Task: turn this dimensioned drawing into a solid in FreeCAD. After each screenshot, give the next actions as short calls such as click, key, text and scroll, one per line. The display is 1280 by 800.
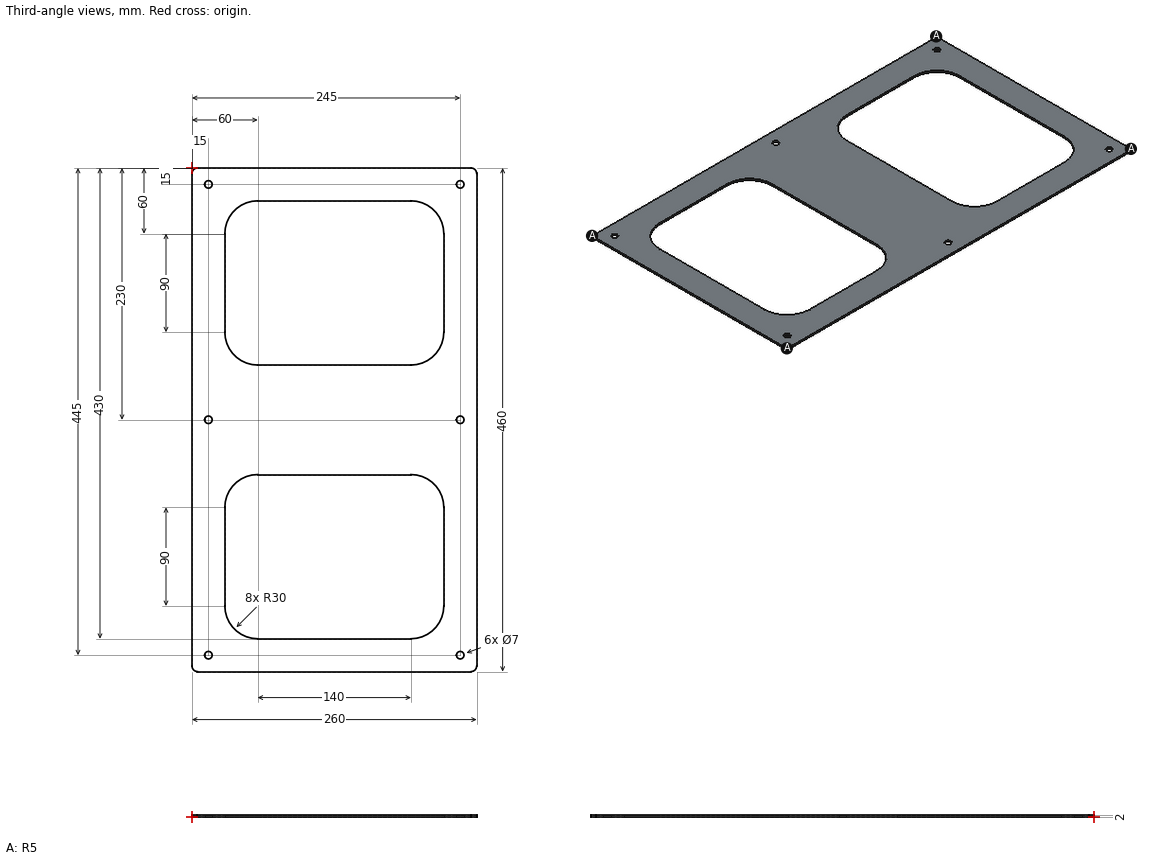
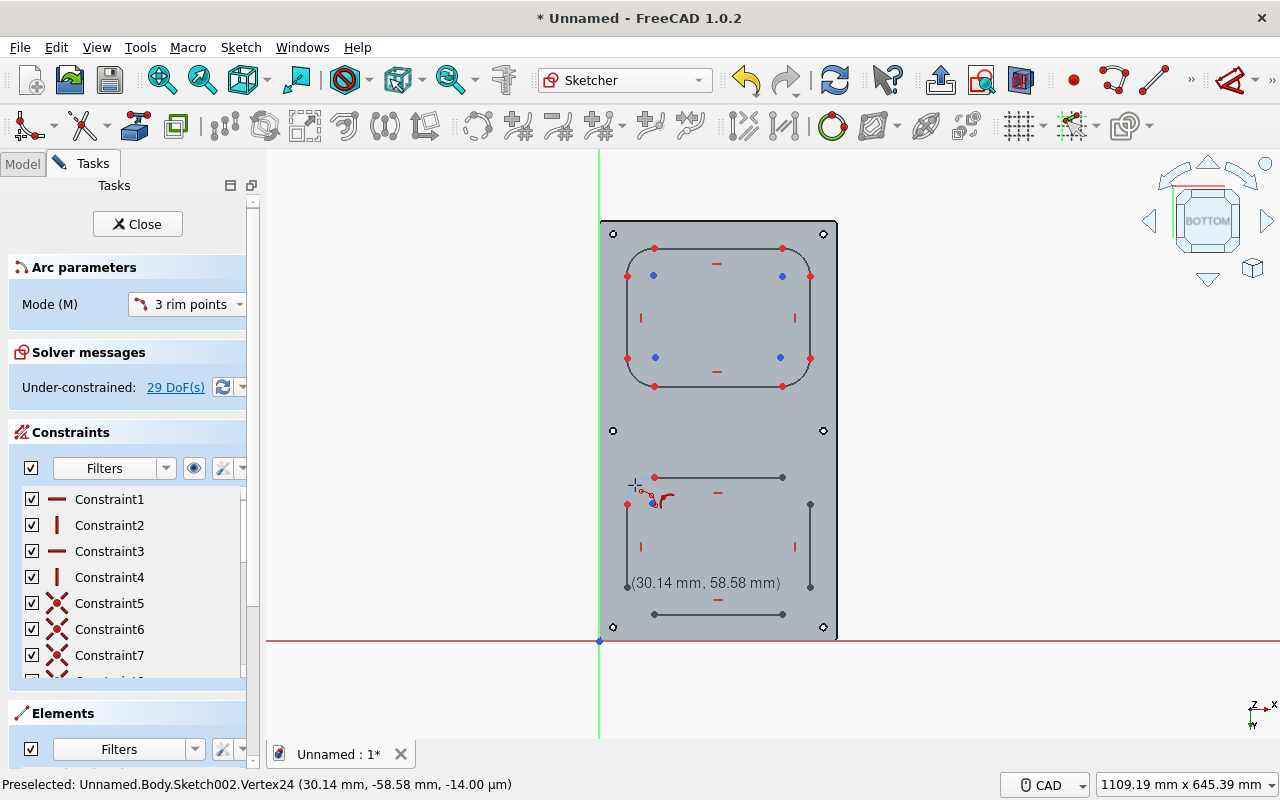
click(654, 615)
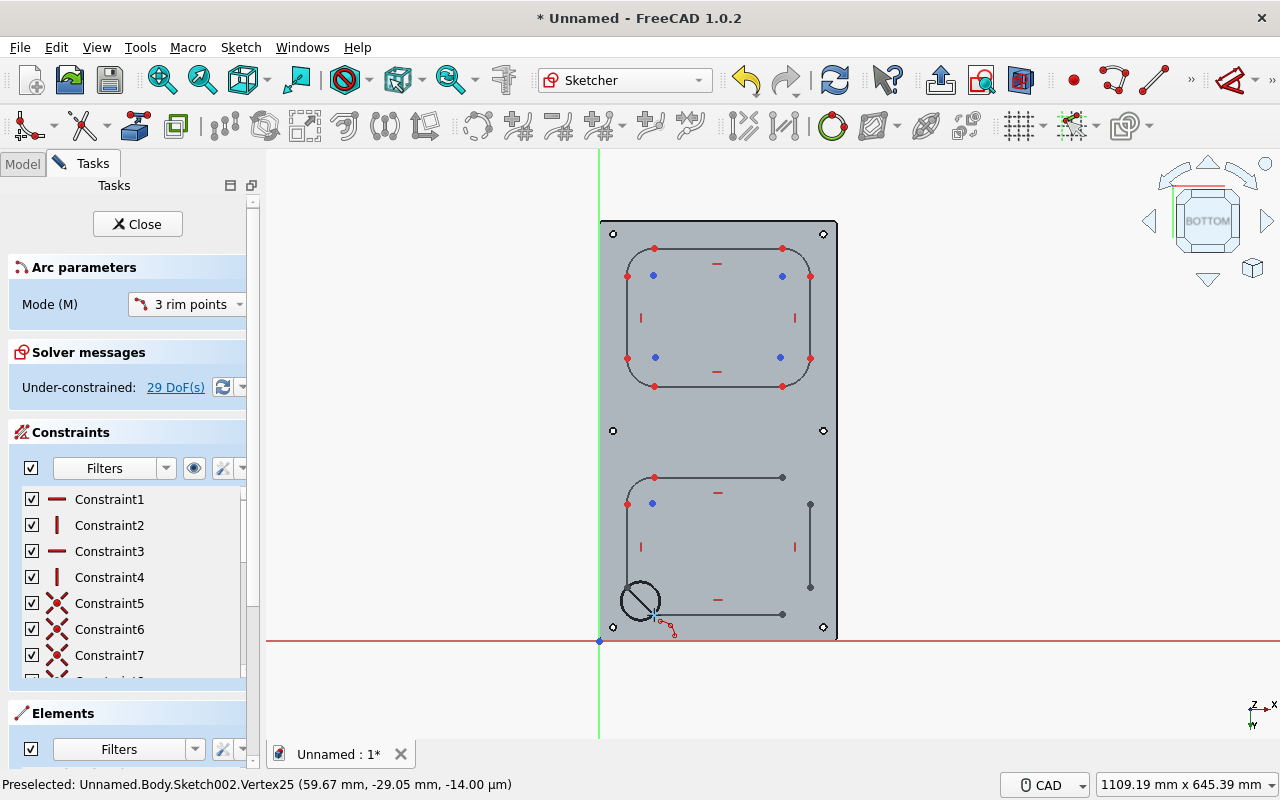
scroll(635, 606, up, 4)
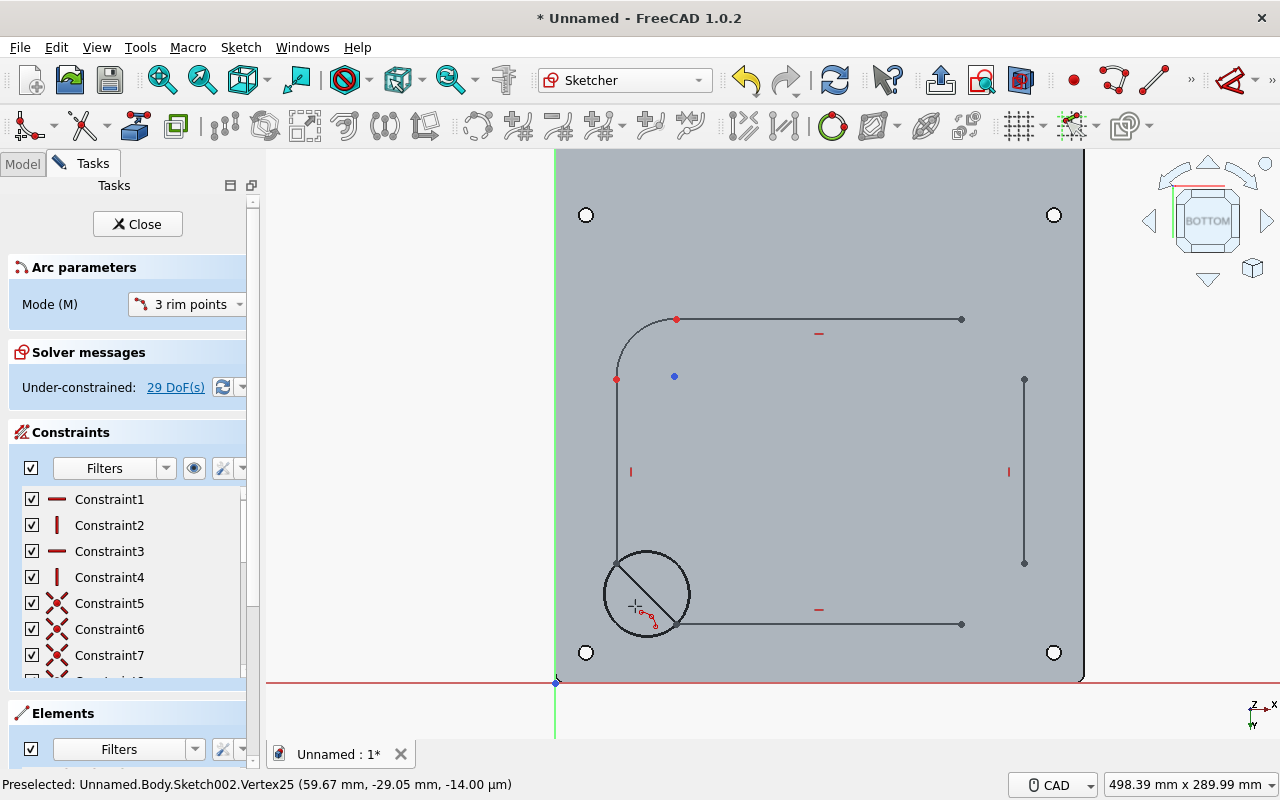
click(634, 604)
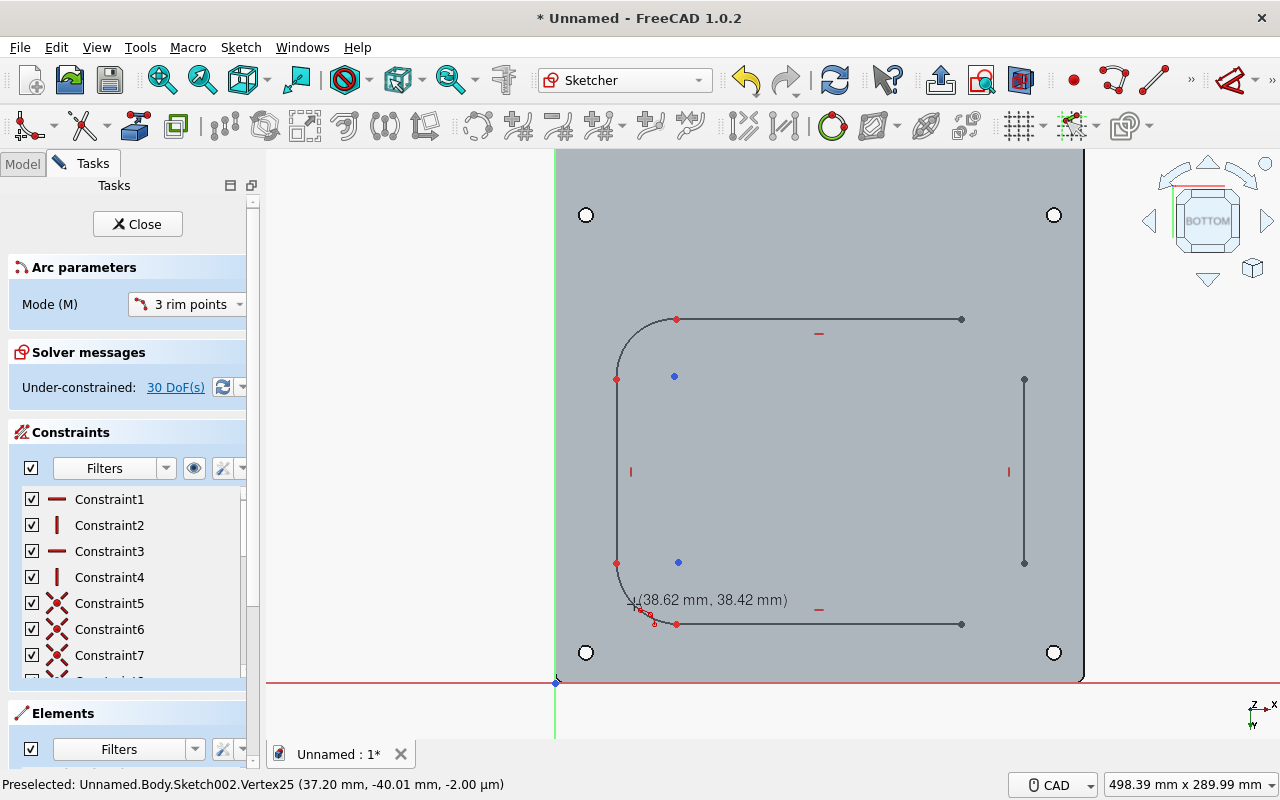
click(962, 624)
click(1024, 564)
click(1006, 604)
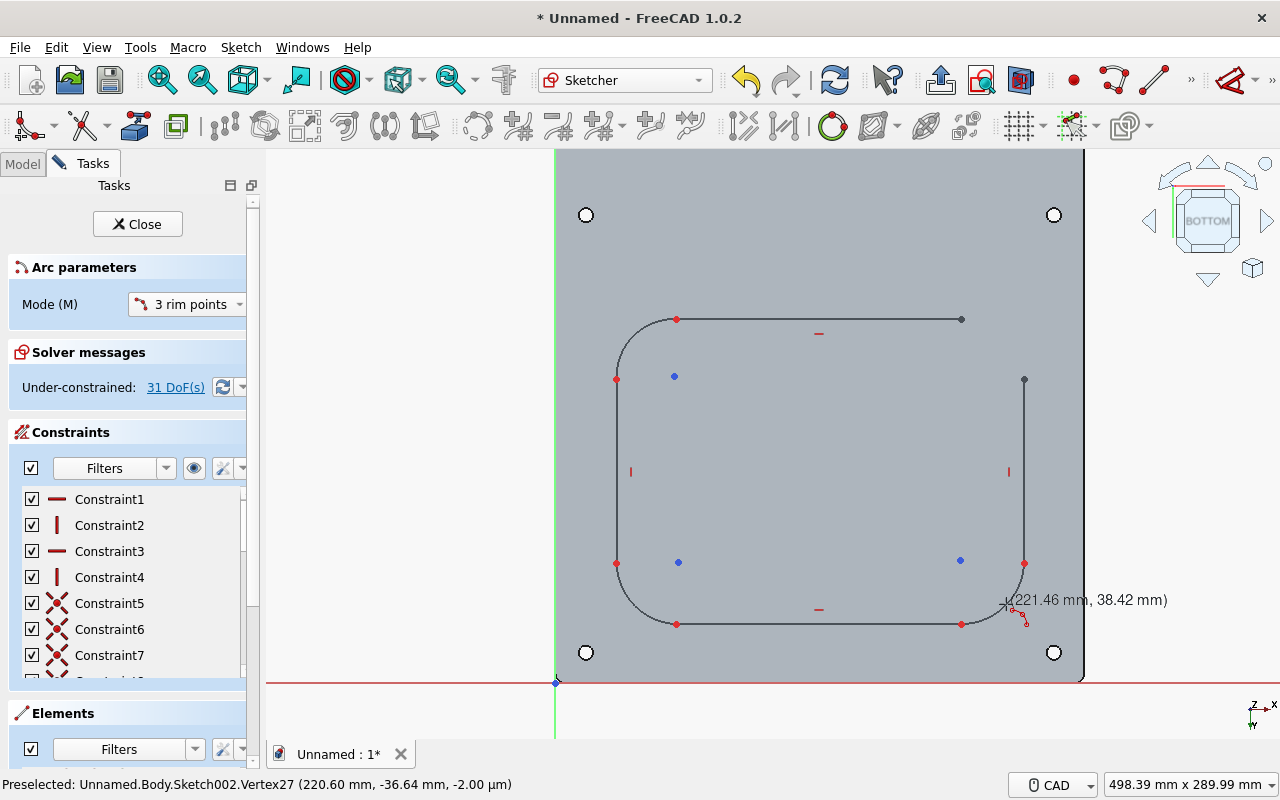
click(1024, 379)
click(962, 319)
click(1006, 335)
key(Escape)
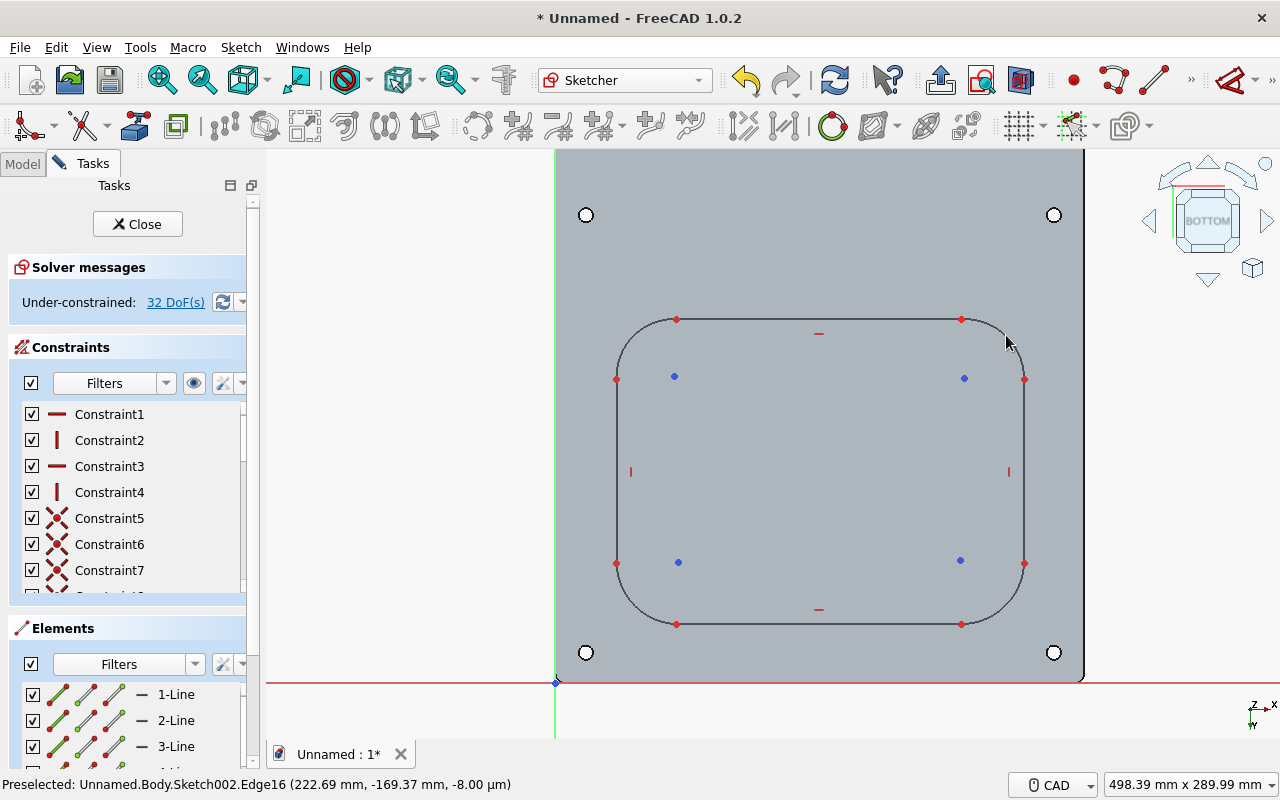
scroll(635, 606, down, 4)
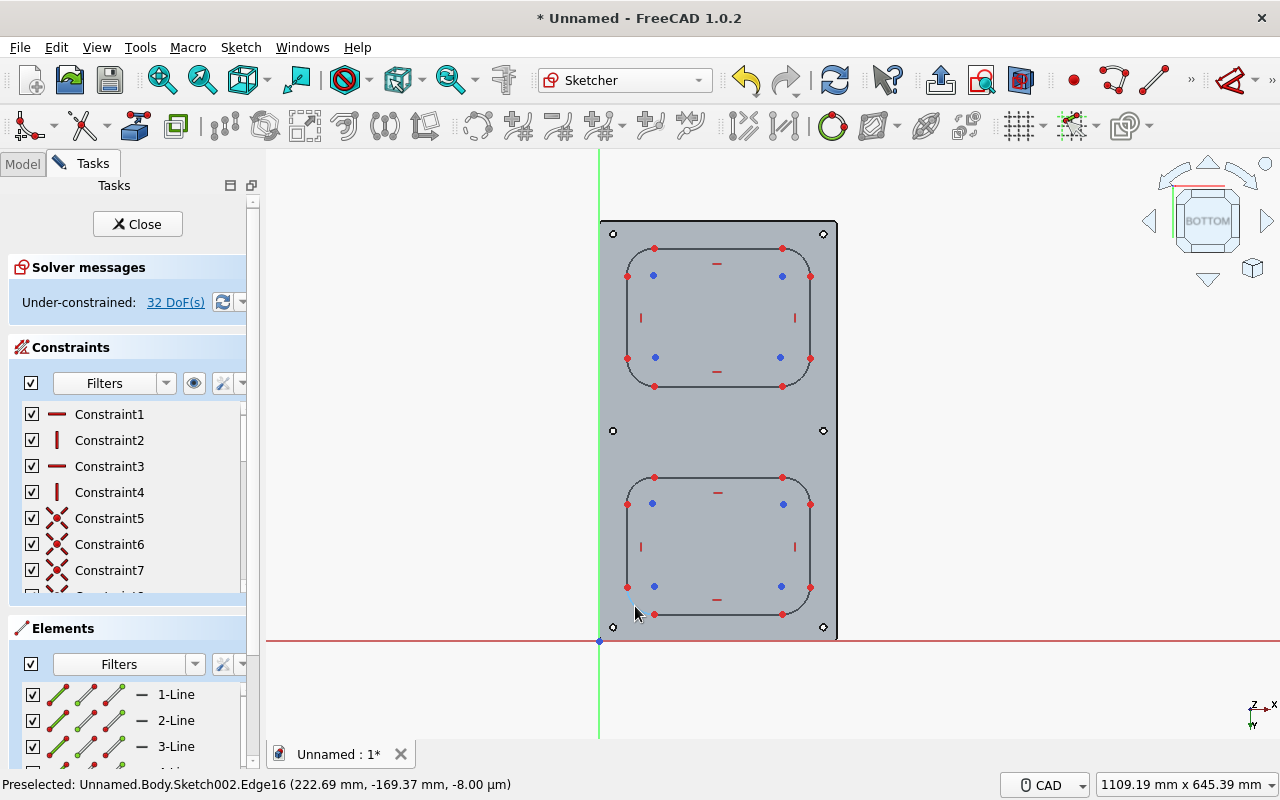
click(744, 249)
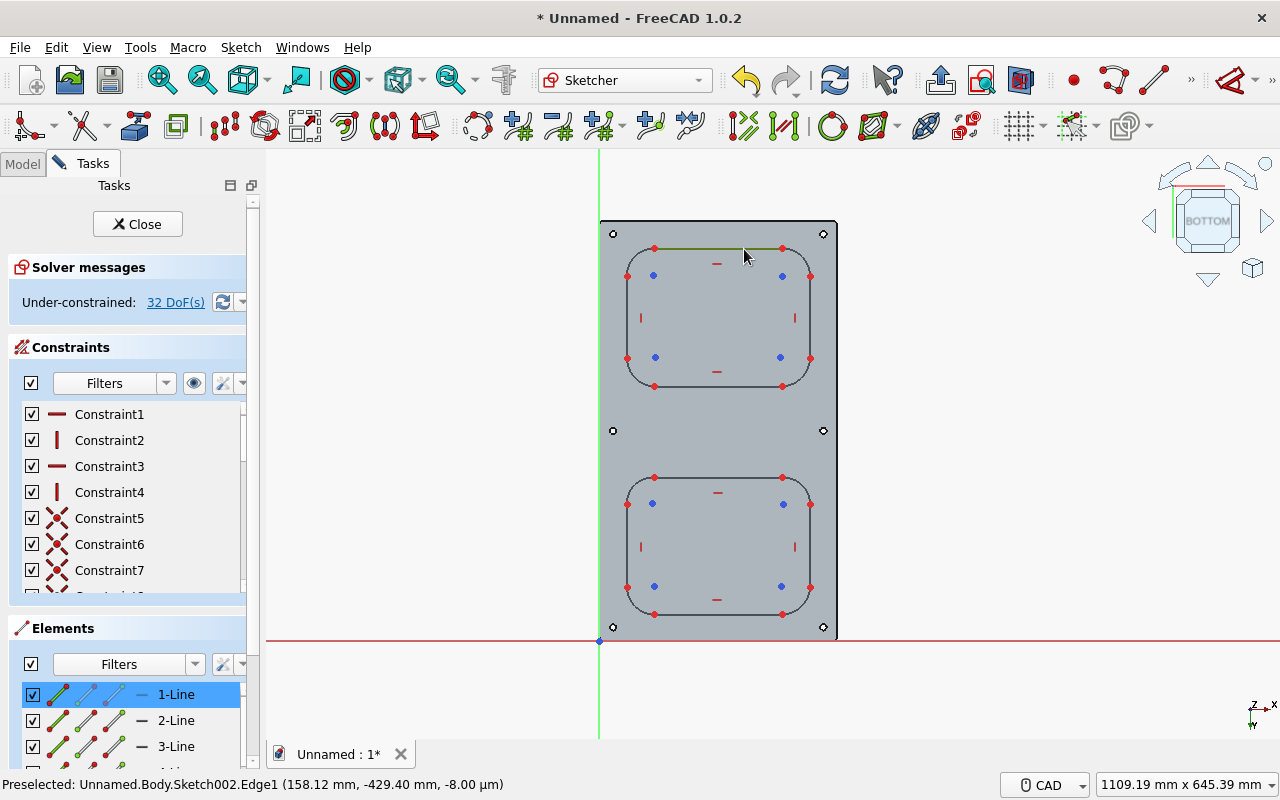
click(641, 252)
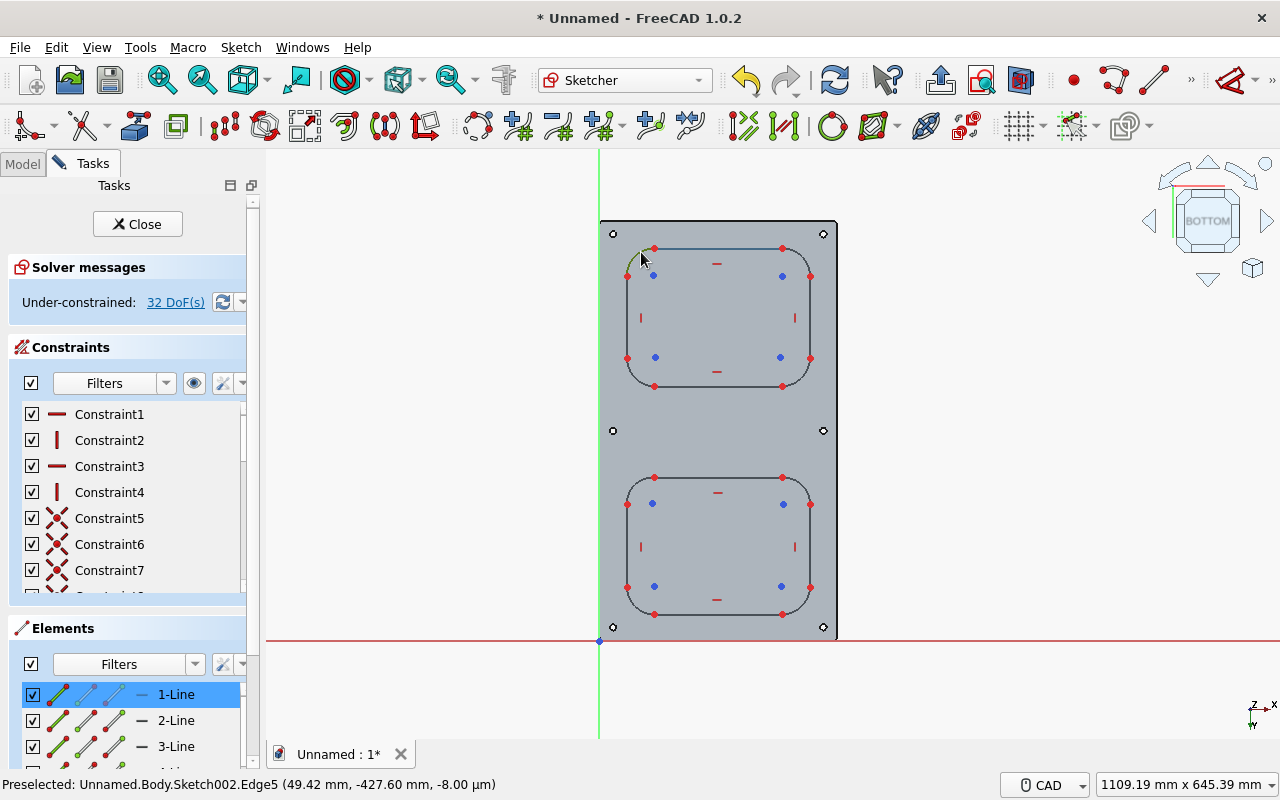
key(t)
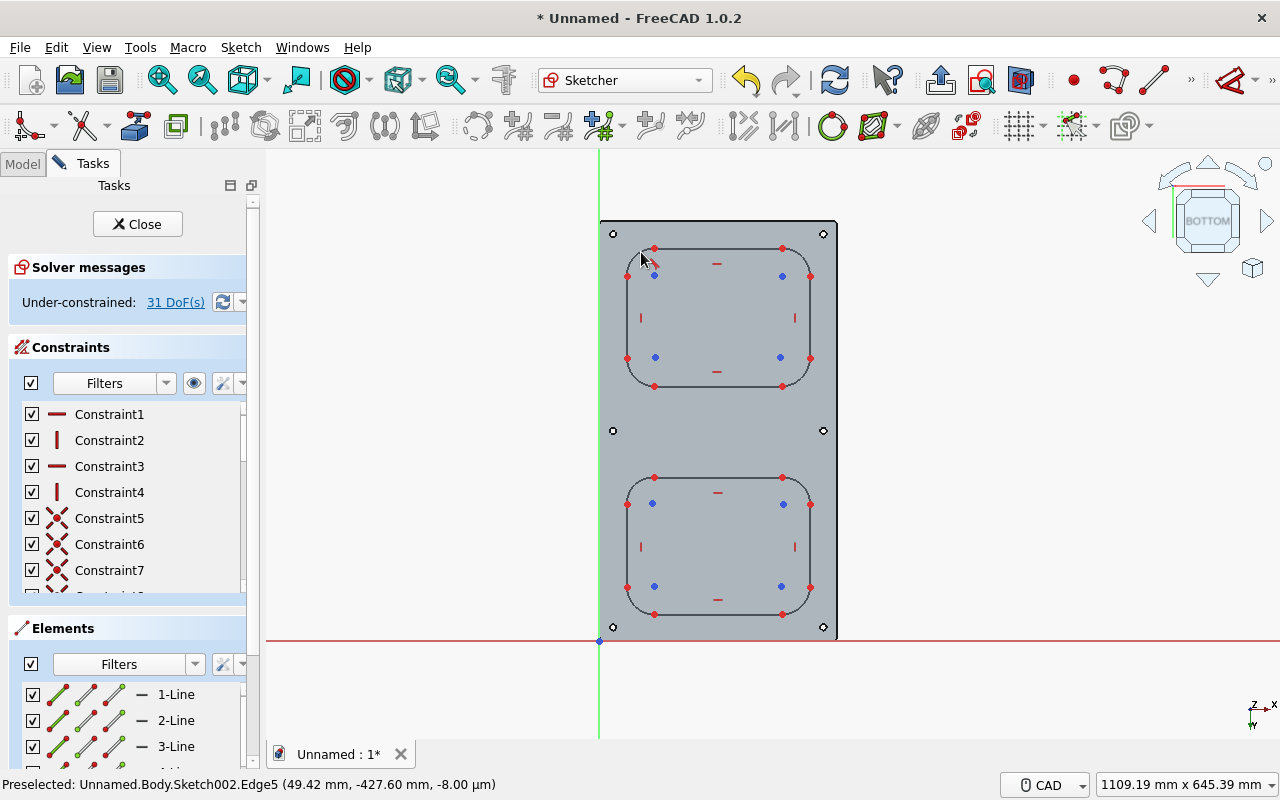
click(744, 249)